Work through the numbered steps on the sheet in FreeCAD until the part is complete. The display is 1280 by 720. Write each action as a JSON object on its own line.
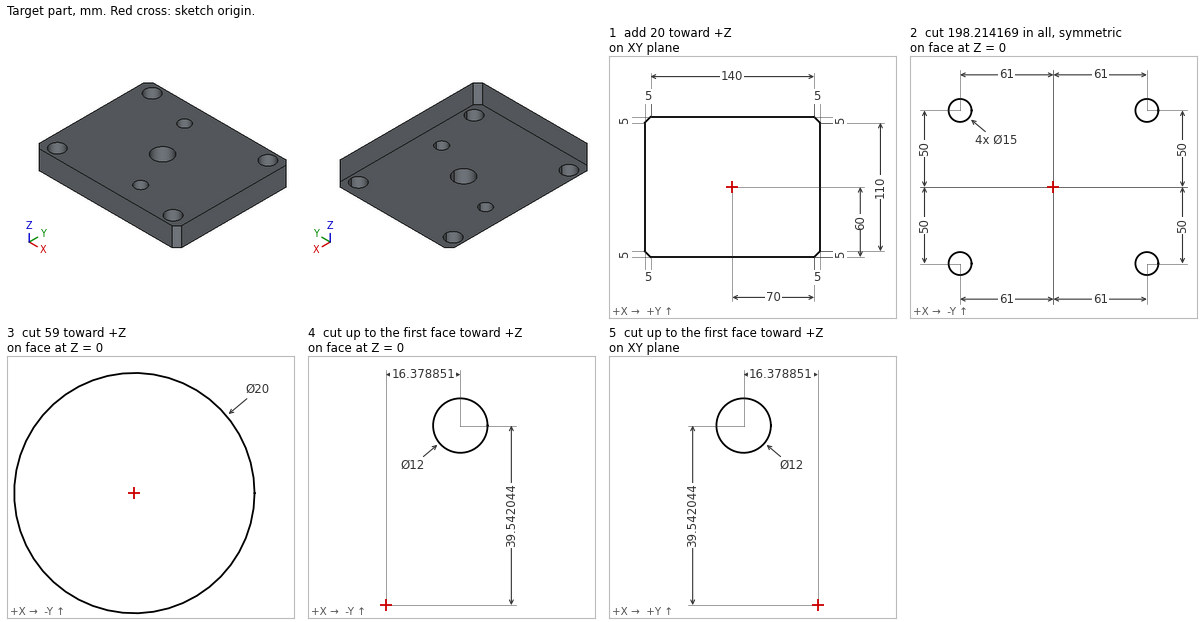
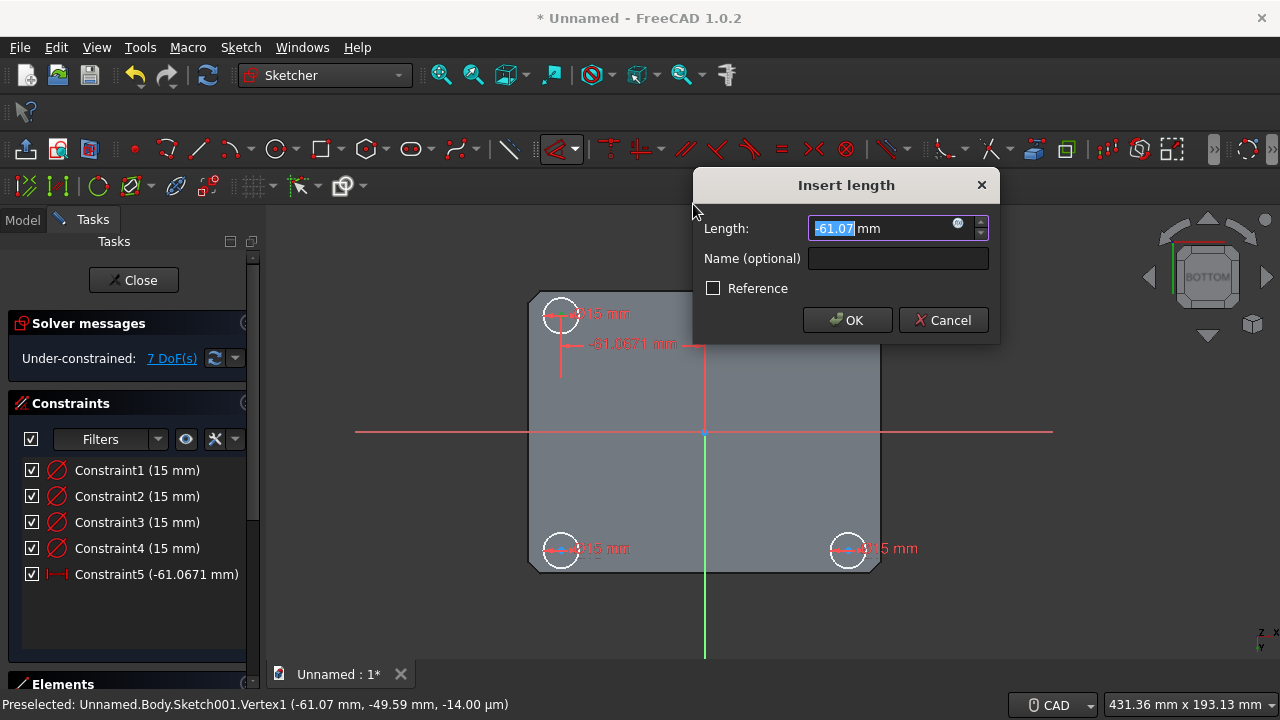
{"action": "type", "text": "-61"}
{"action": "key", "text": "Return"}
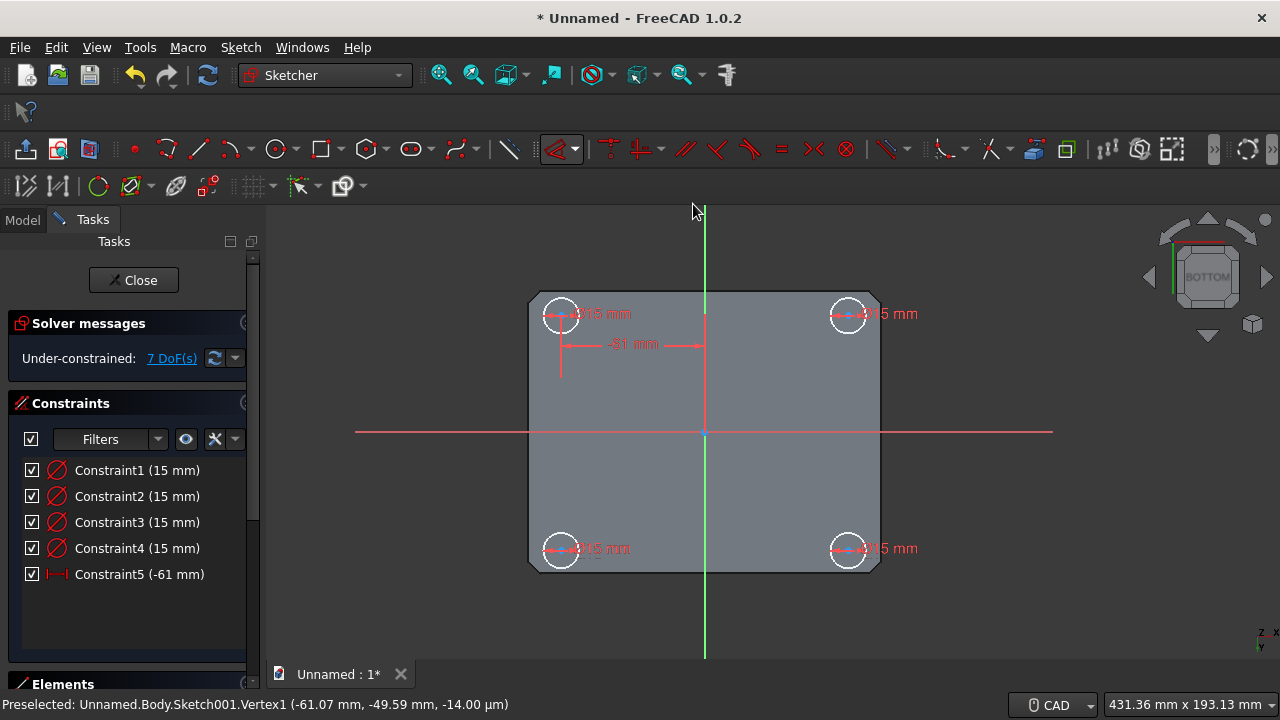
{"action": "left_click", "coordinate": [561, 316]}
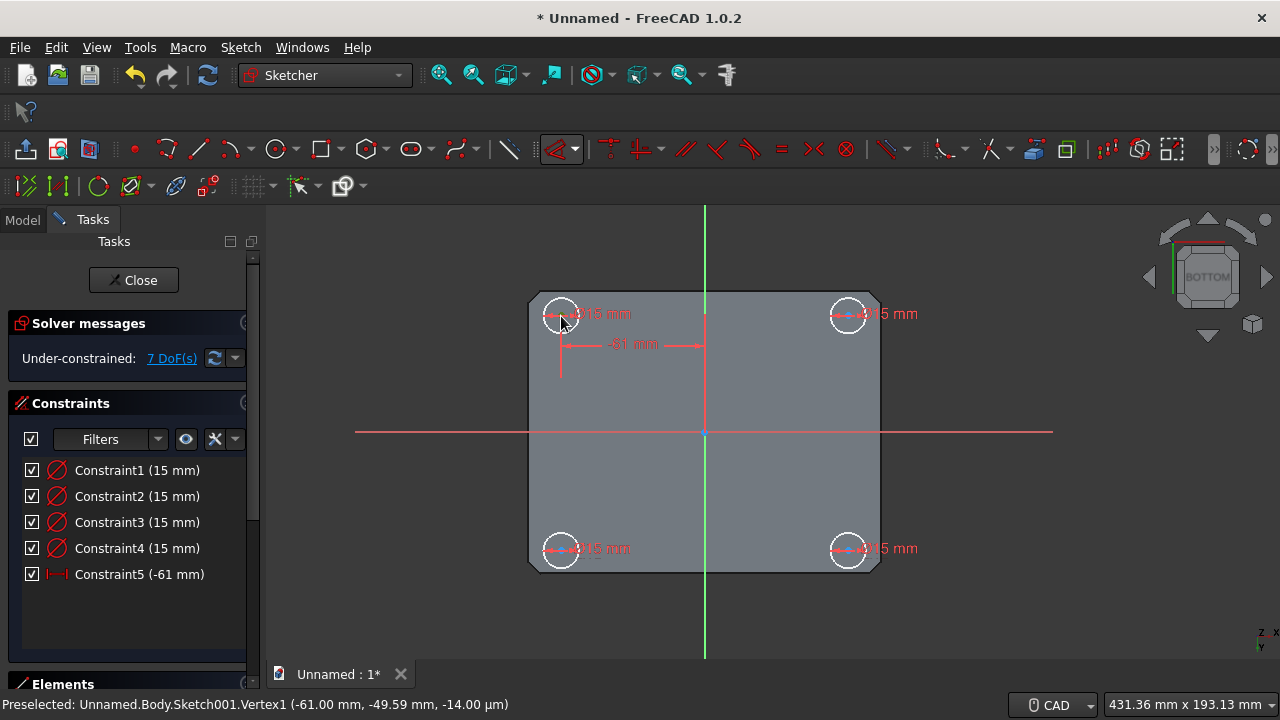
{"action": "key", "text": "i"}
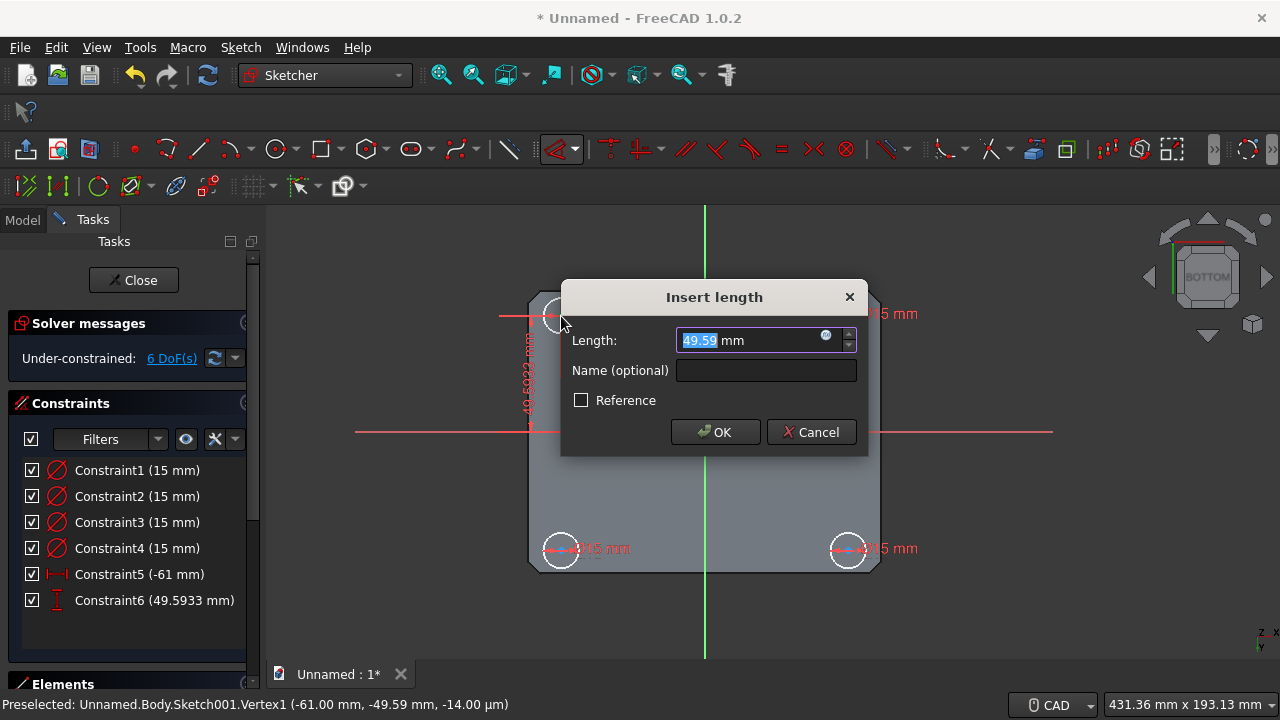
{"action": "type", "text": "50"}
{"action": "key", "text": "Return"}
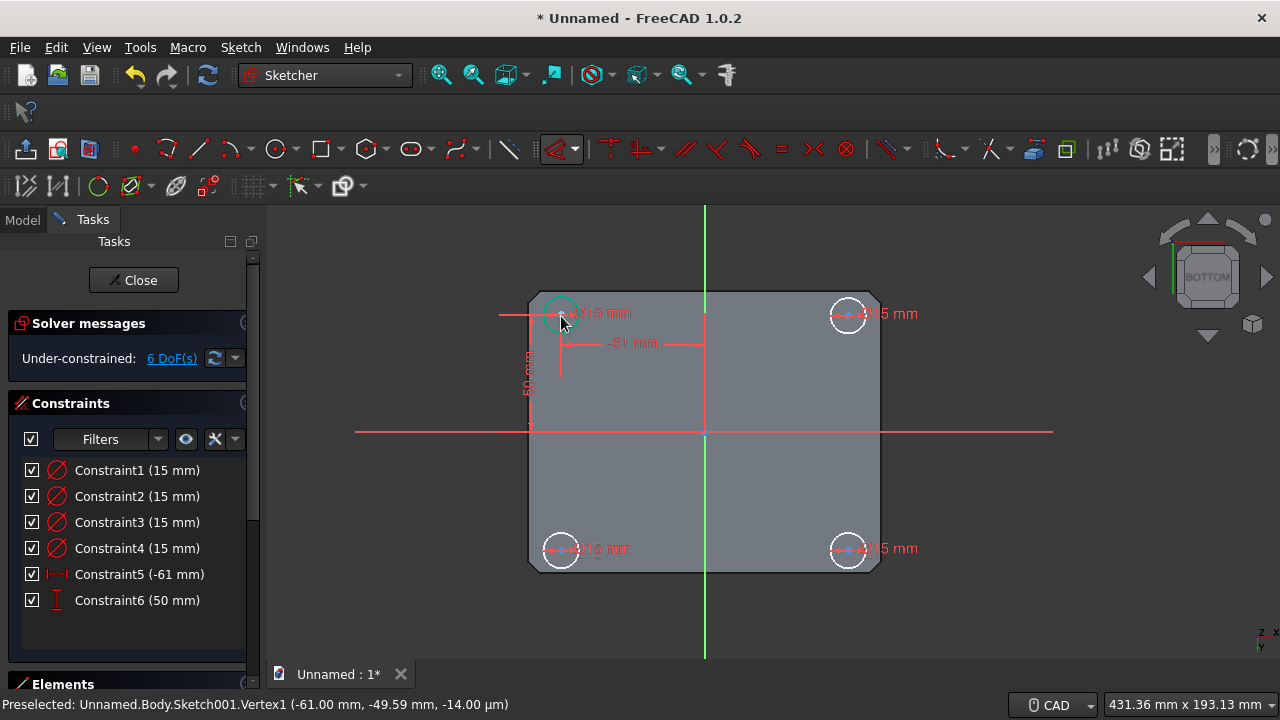
{"action": "left_click", "coordinate": [561, 551]}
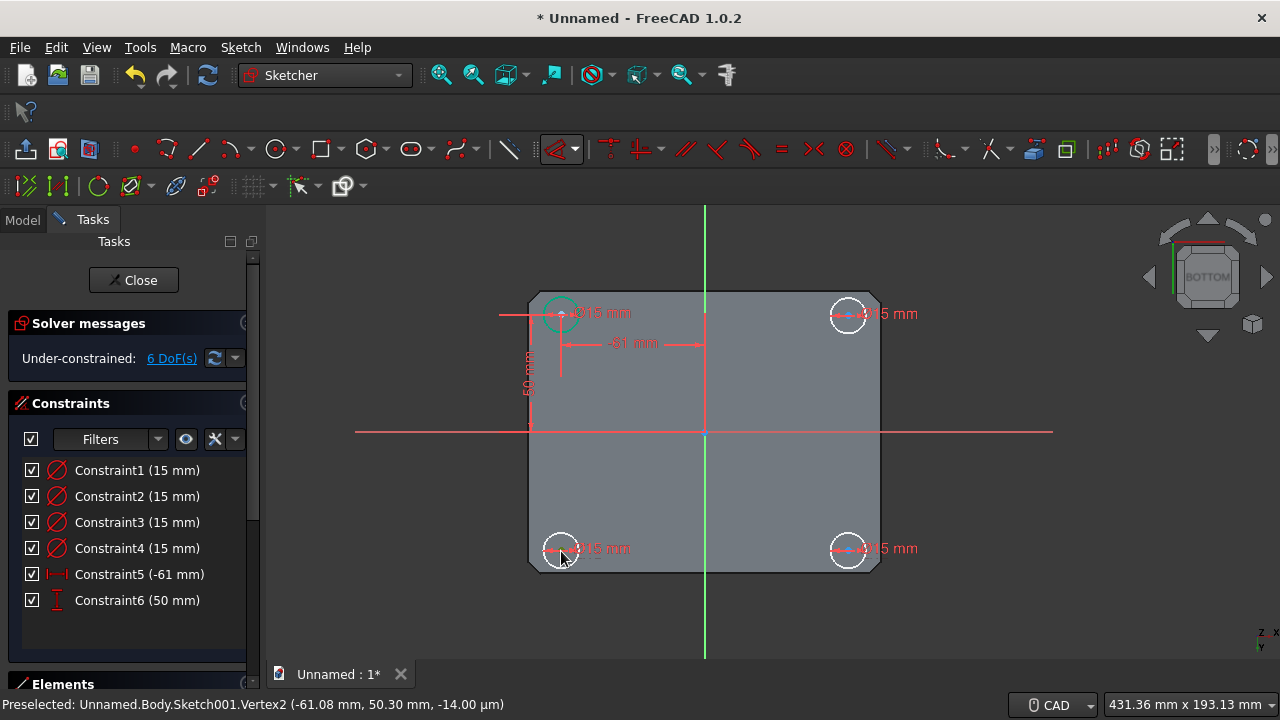
{"action": "key", "text": "l"}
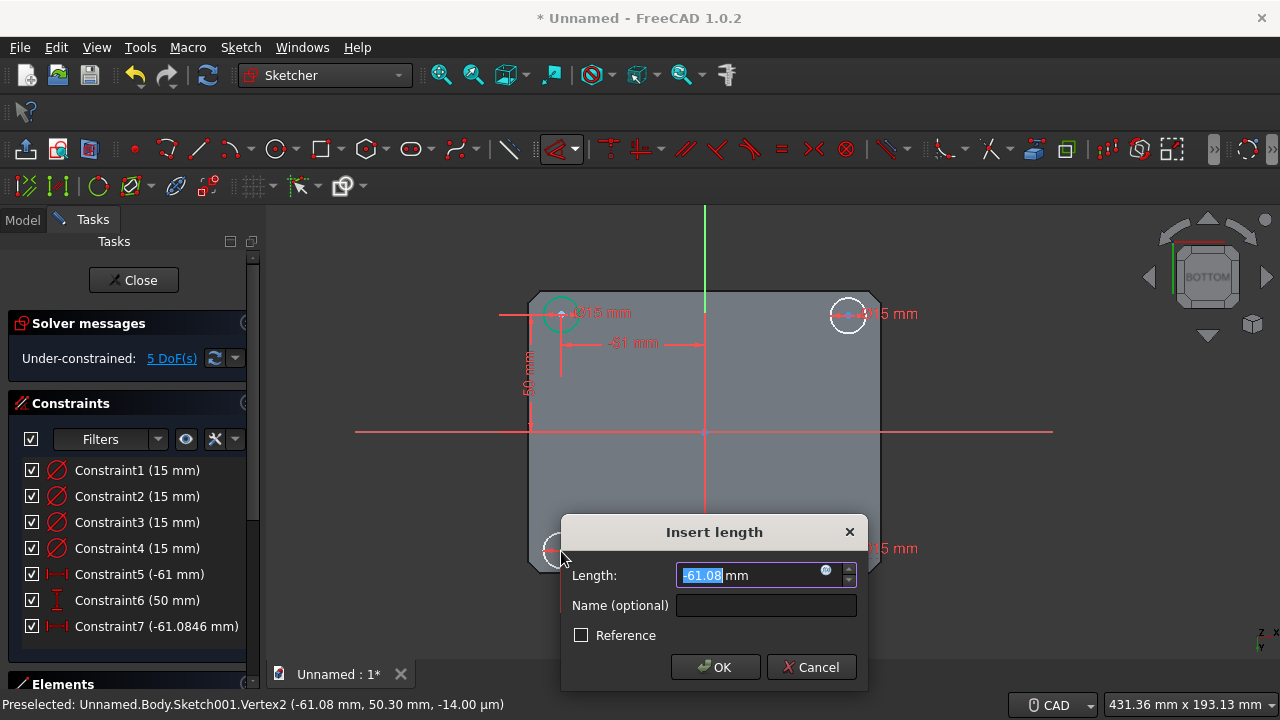
{"action": "type", "text": "-61"}
{"action": "key", "text": "Return"}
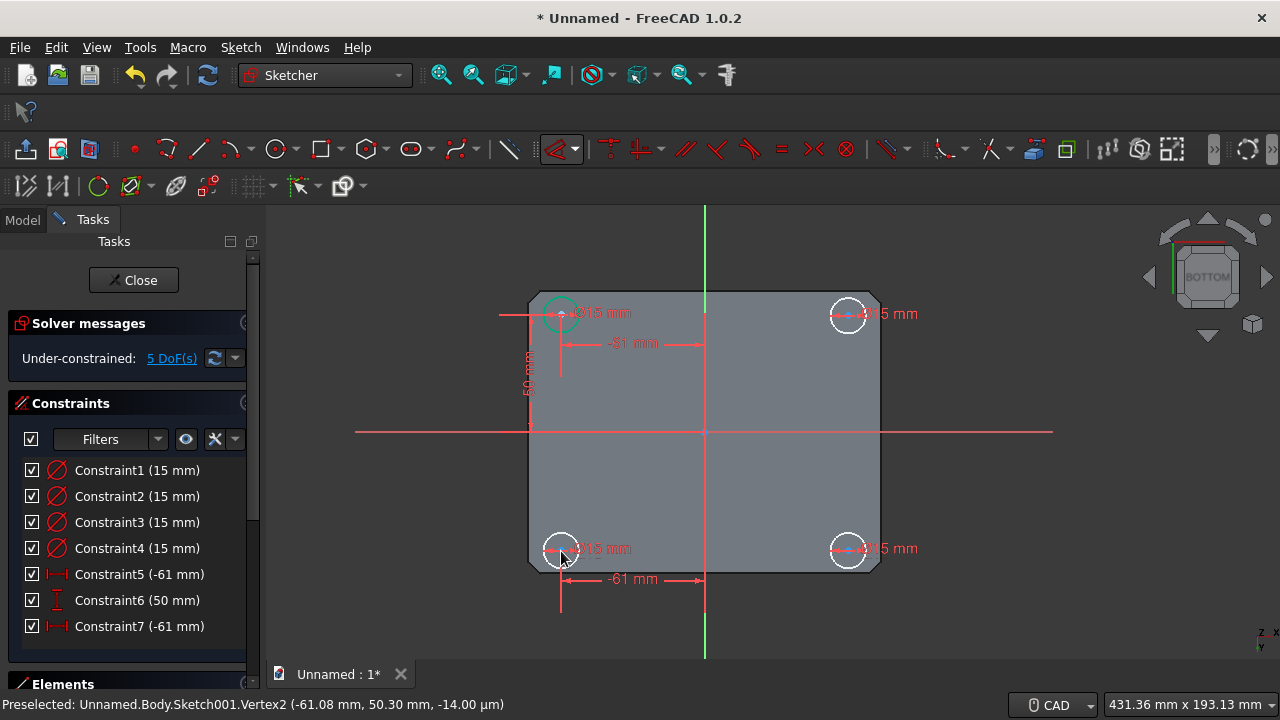
{"action": "left_click", "coordinate": [561, 551]}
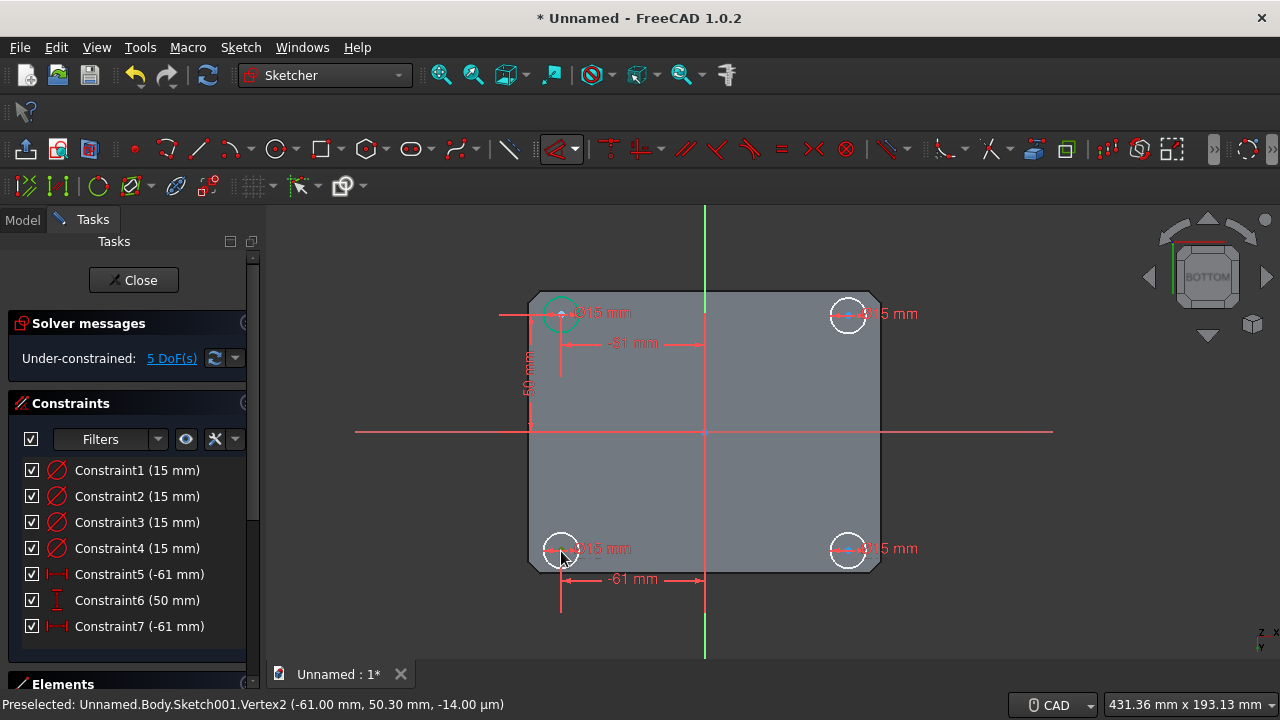
{"action": "left_click", "coordinate": [578, 150]}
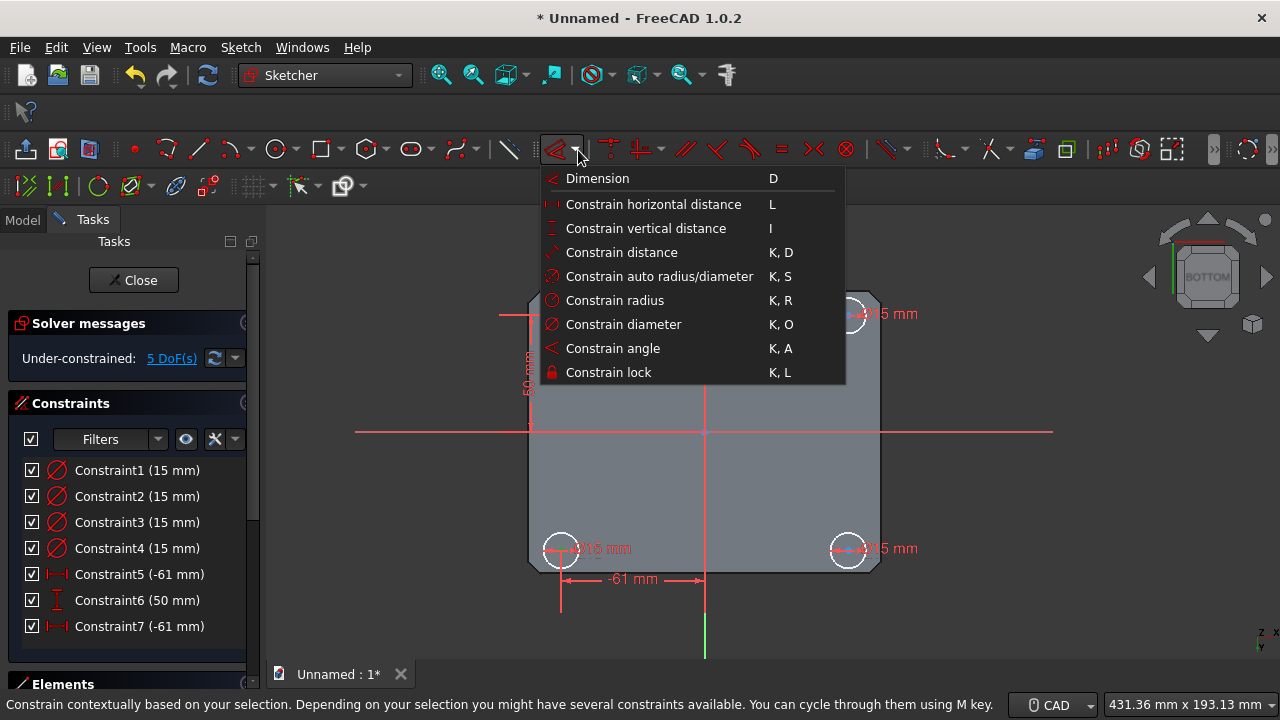
{"action": "left_click", "coordinate": [693, 228]}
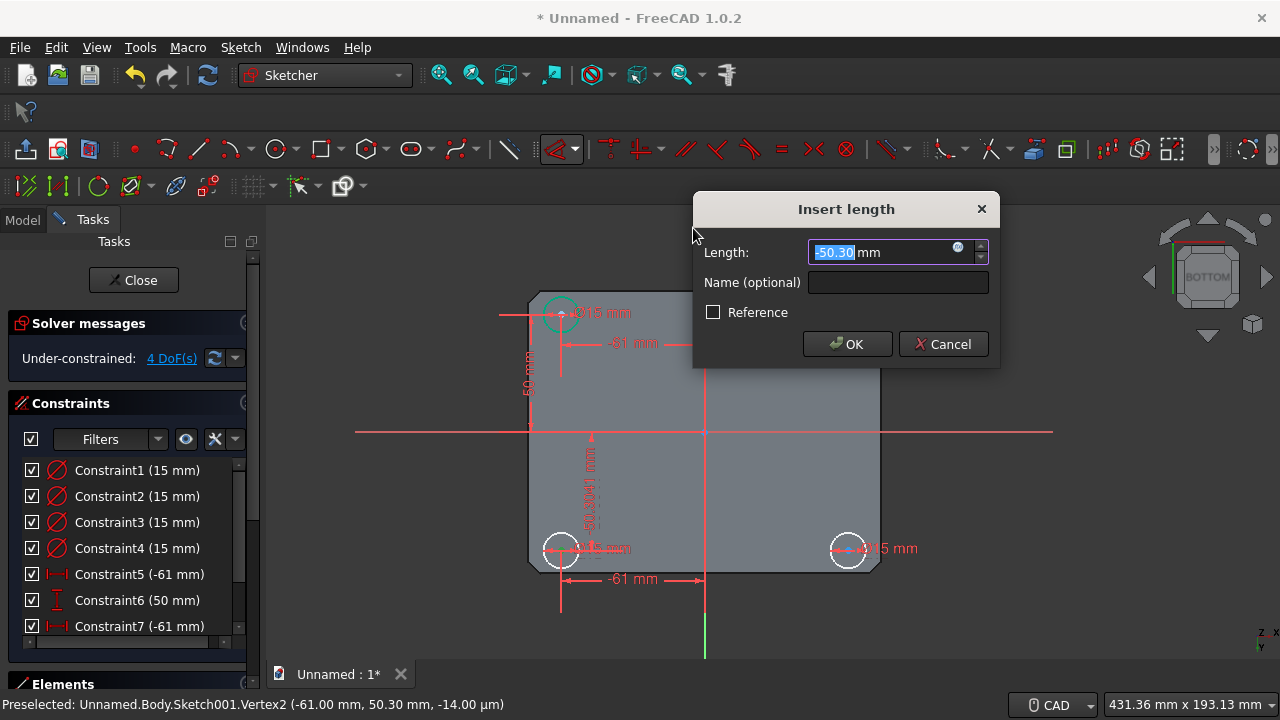
{"action": "type", "text": "-50"}
{"action": "key", "text": "Return"}